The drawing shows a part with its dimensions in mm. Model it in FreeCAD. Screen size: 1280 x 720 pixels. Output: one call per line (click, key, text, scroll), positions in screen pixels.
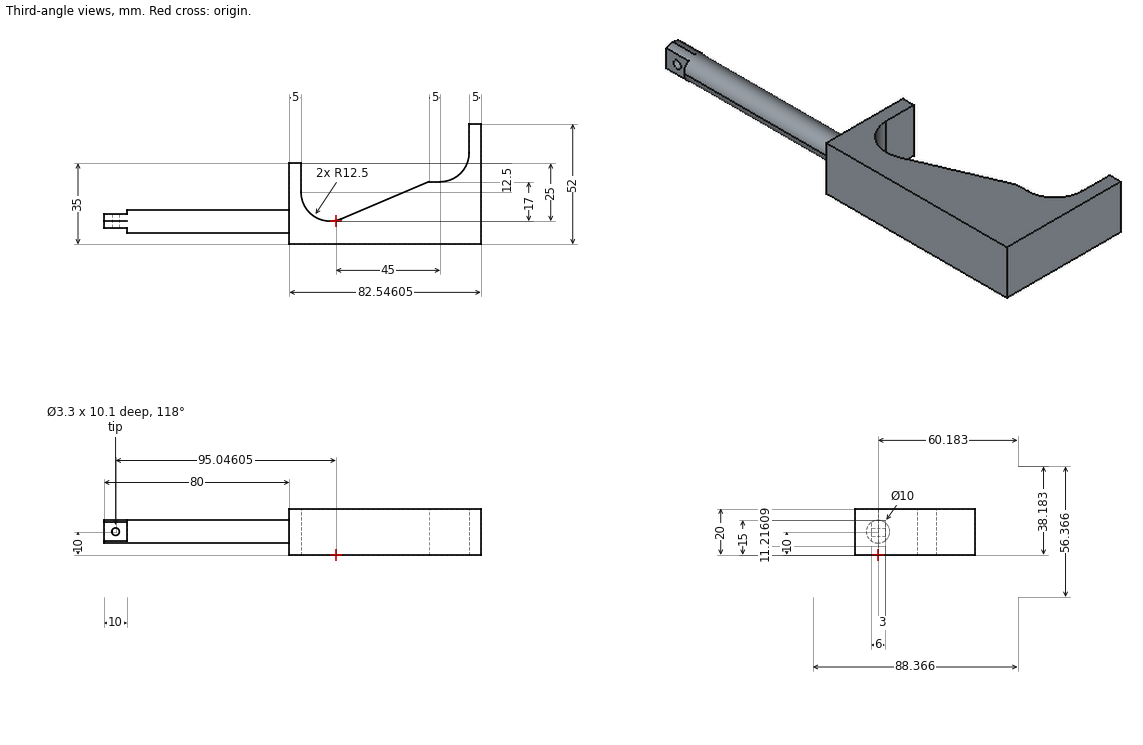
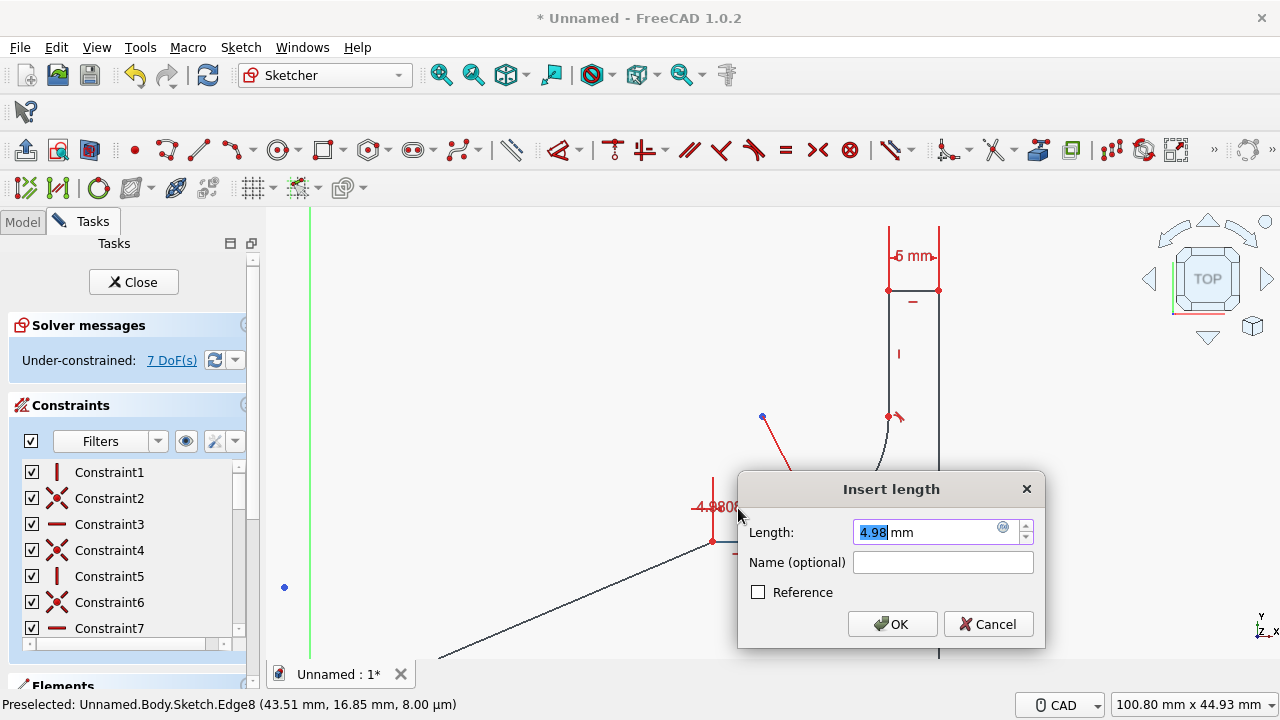
text(5)
key(Return)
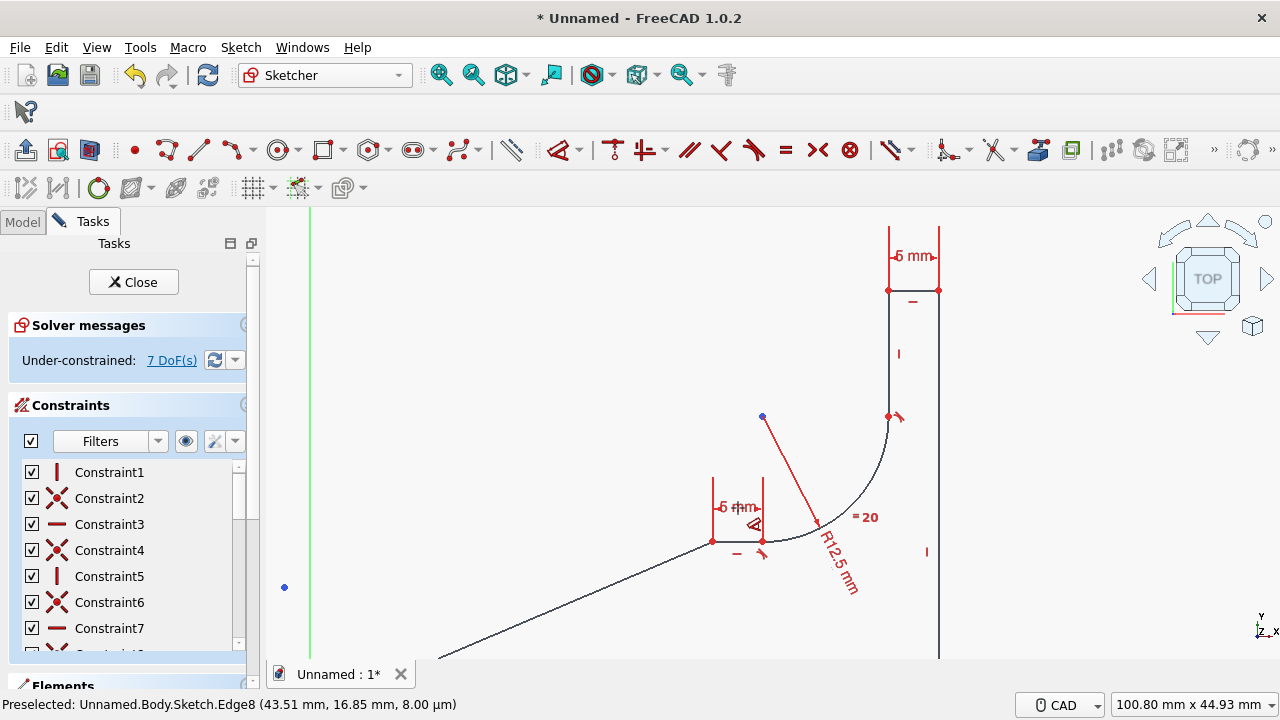
scroll(924, 290, down, 3)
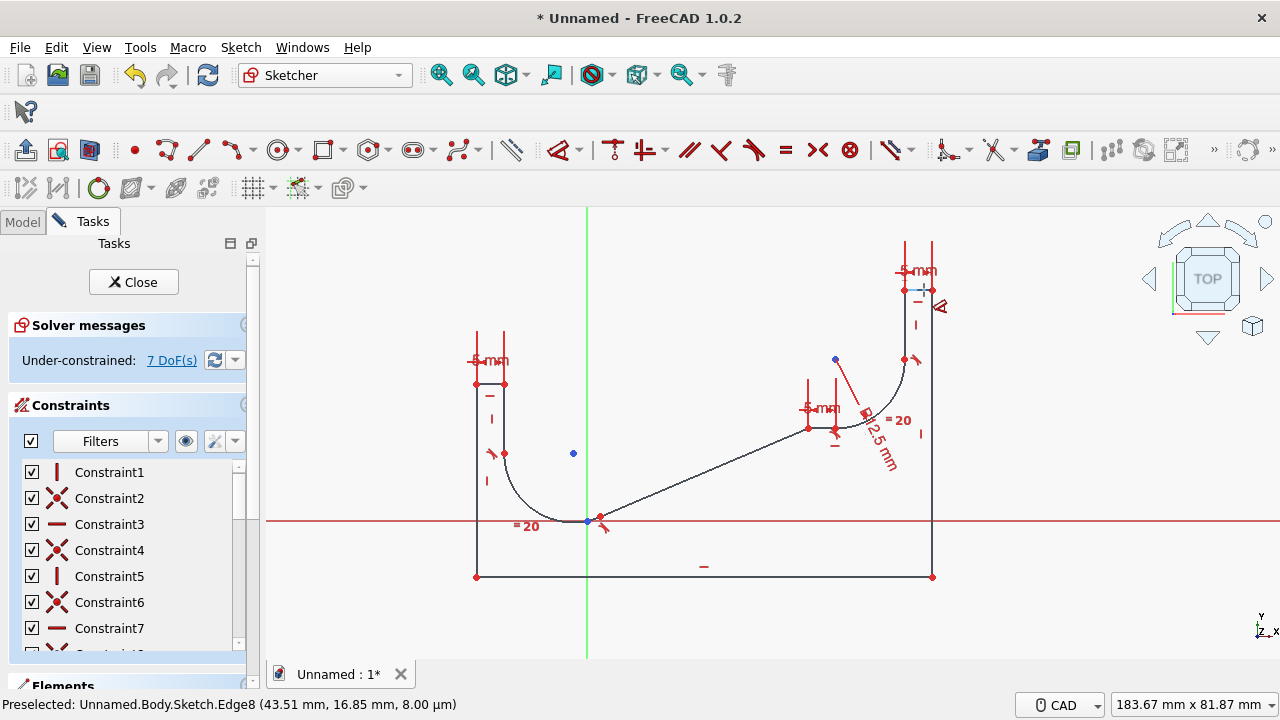
click(477, 442)
click(443, 481)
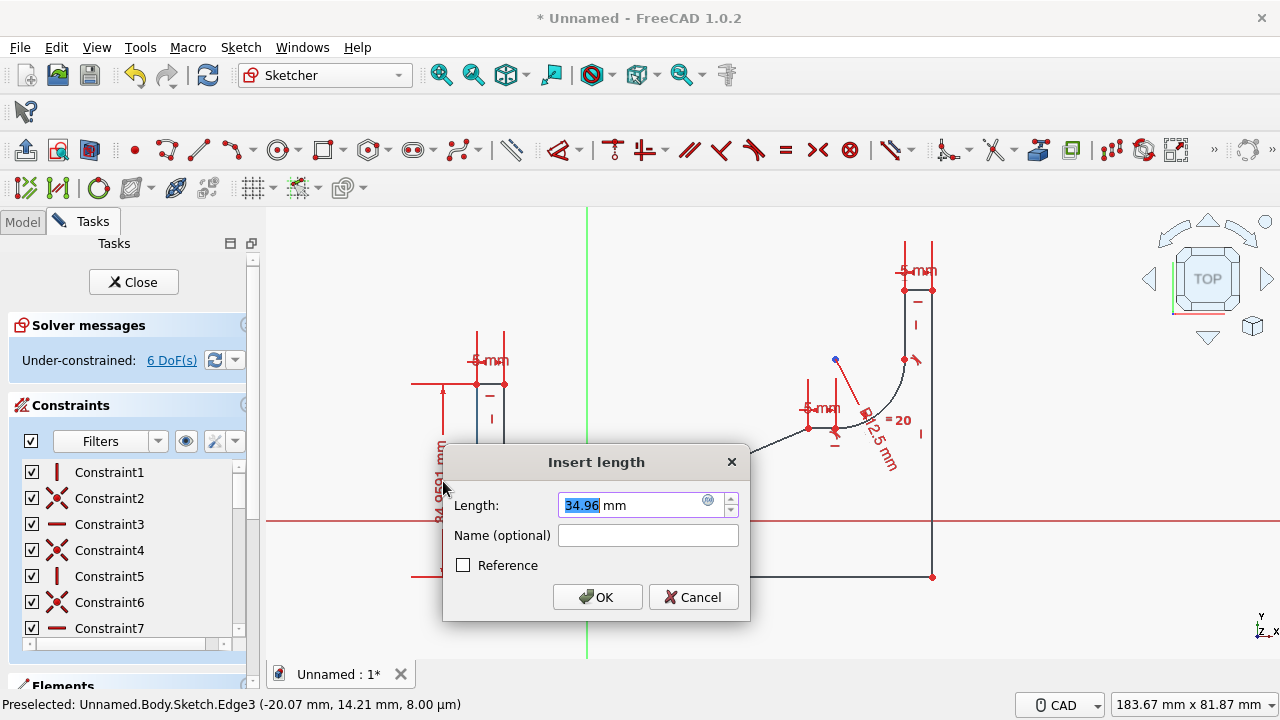
text(35)
key(Return)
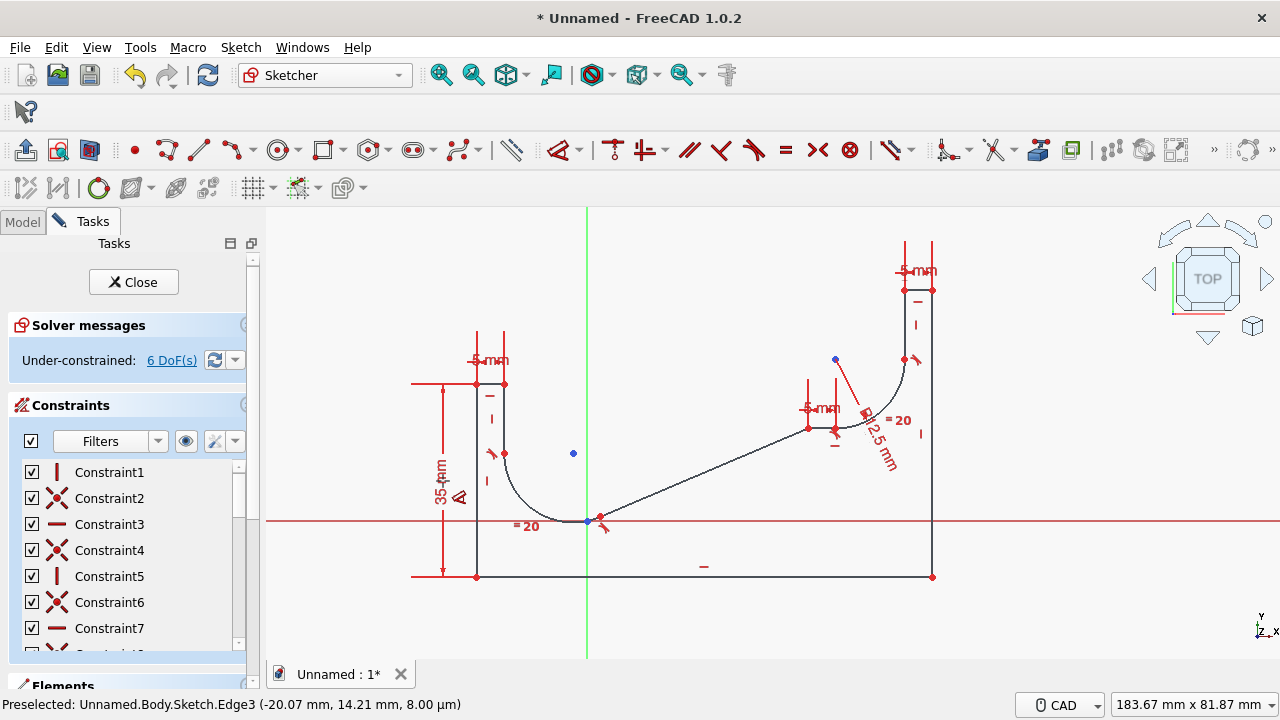
click(932, 491)
click(966, 434)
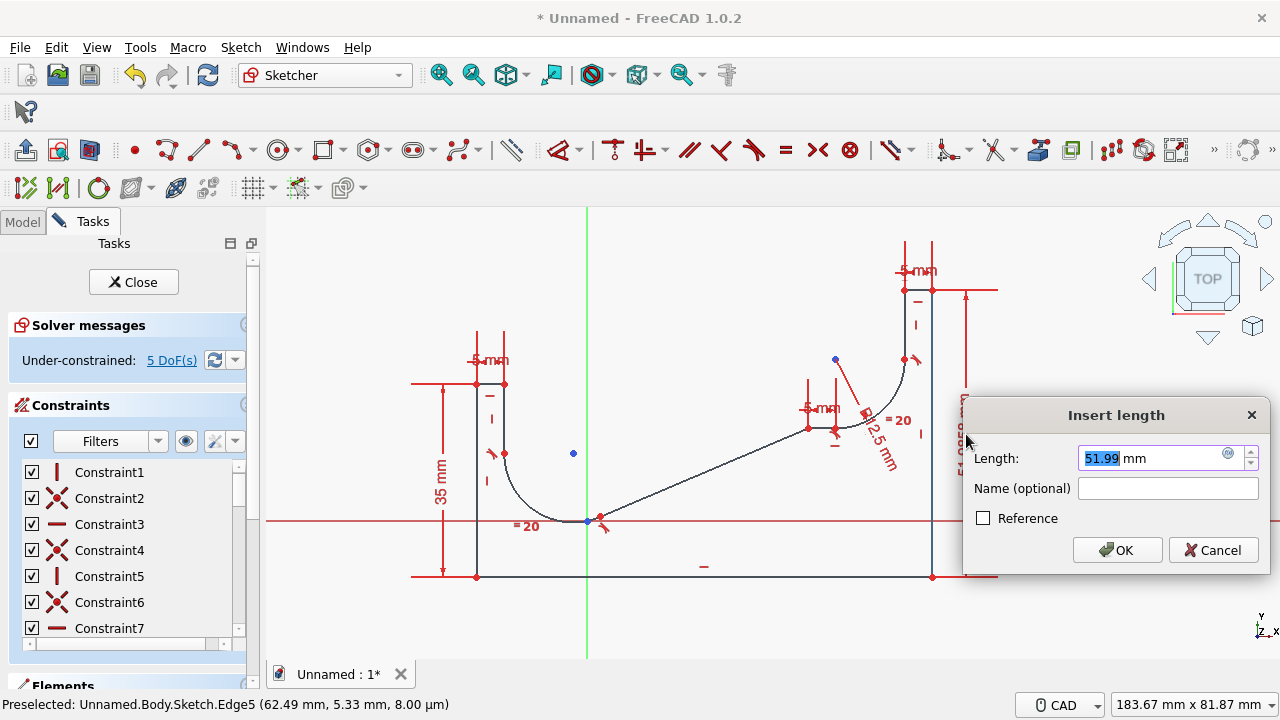
text(52)
key(Return)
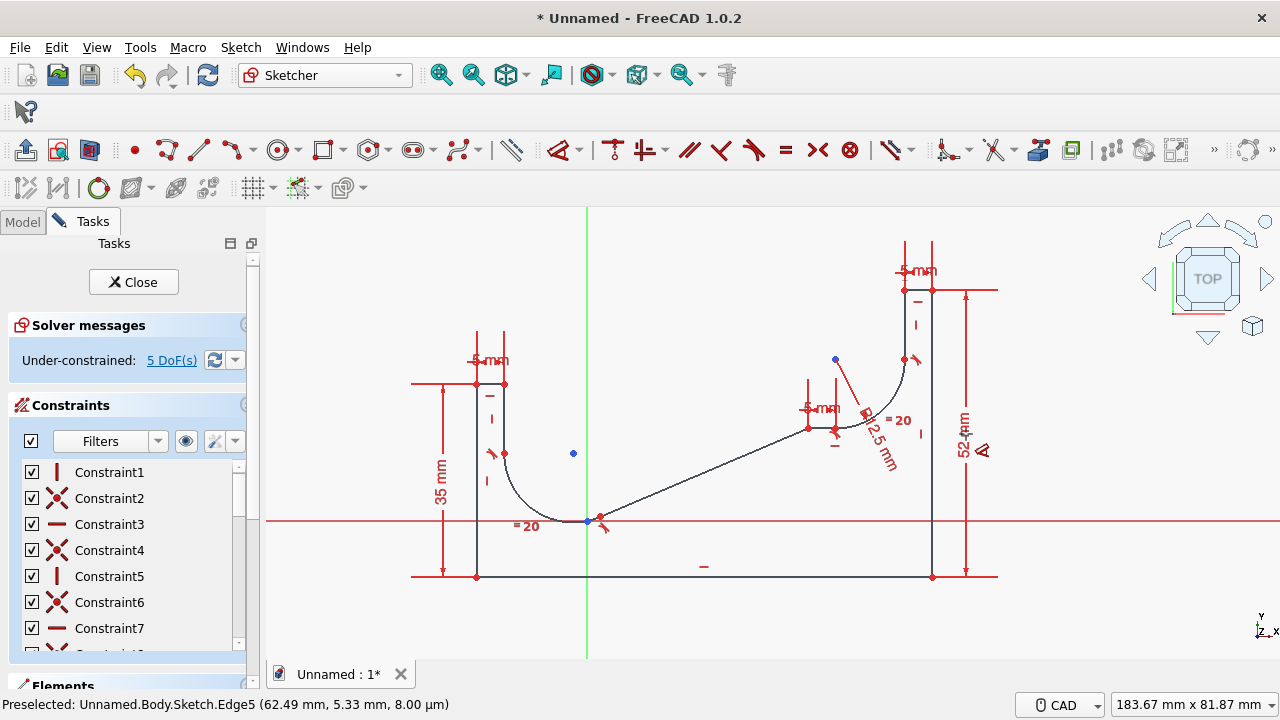
click(504, 384)
click(621, 453)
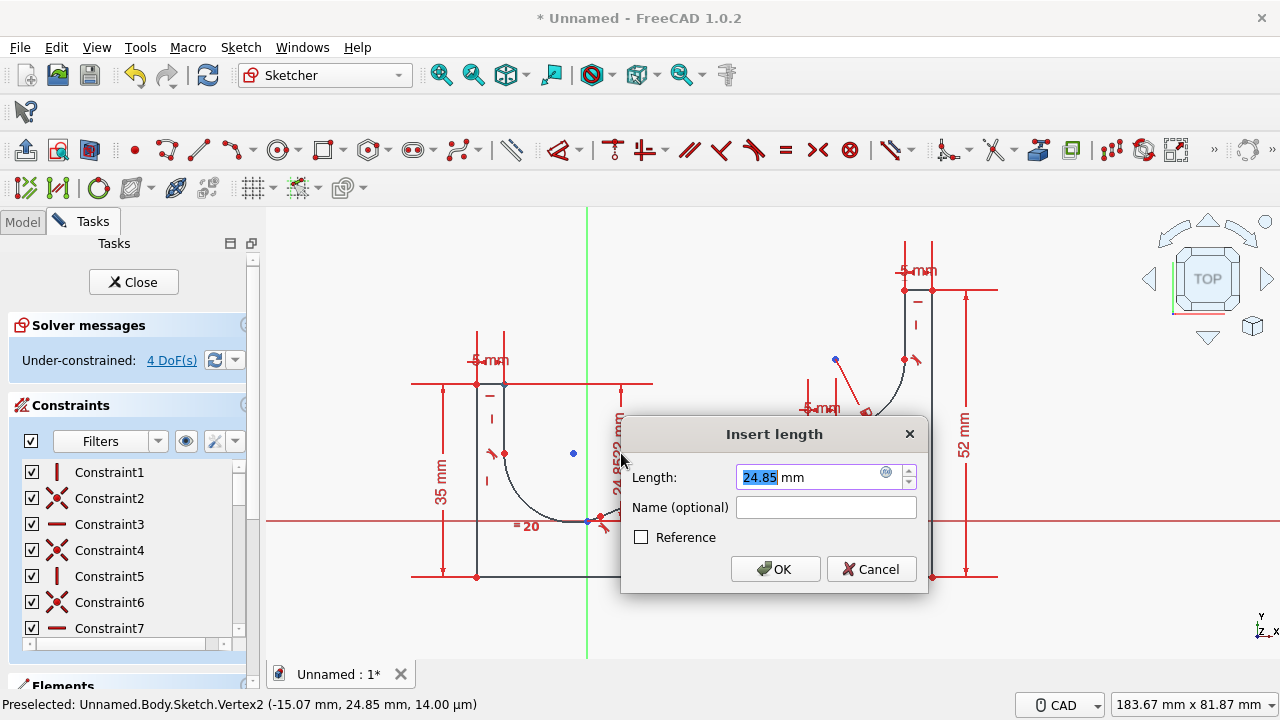
text(25)
key(Return)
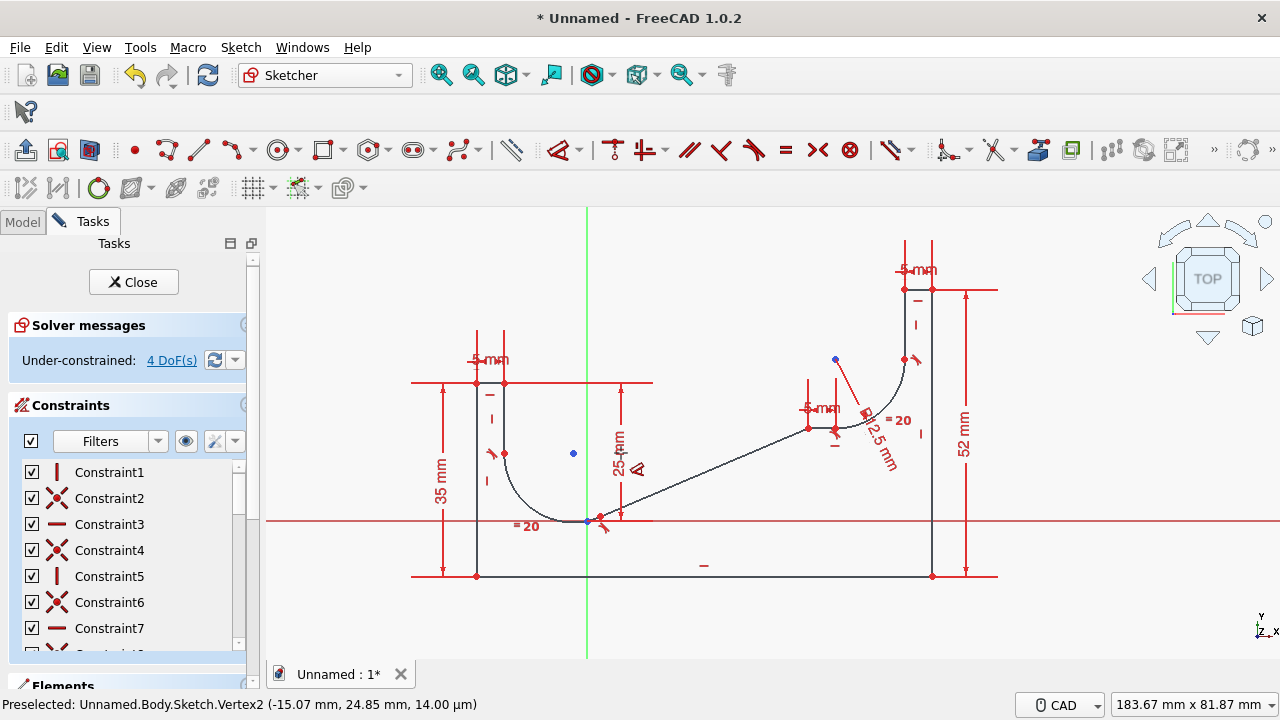
click(836, 428)
click(712, 555)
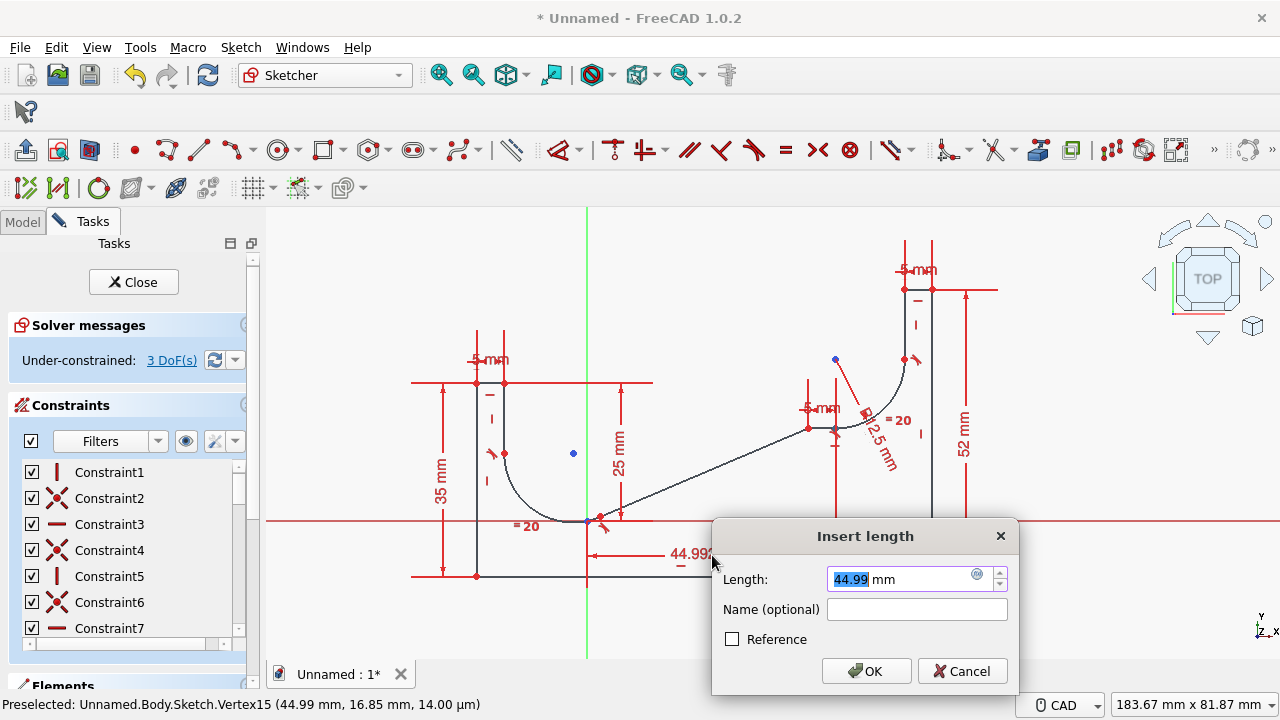
text(45)
key(Return)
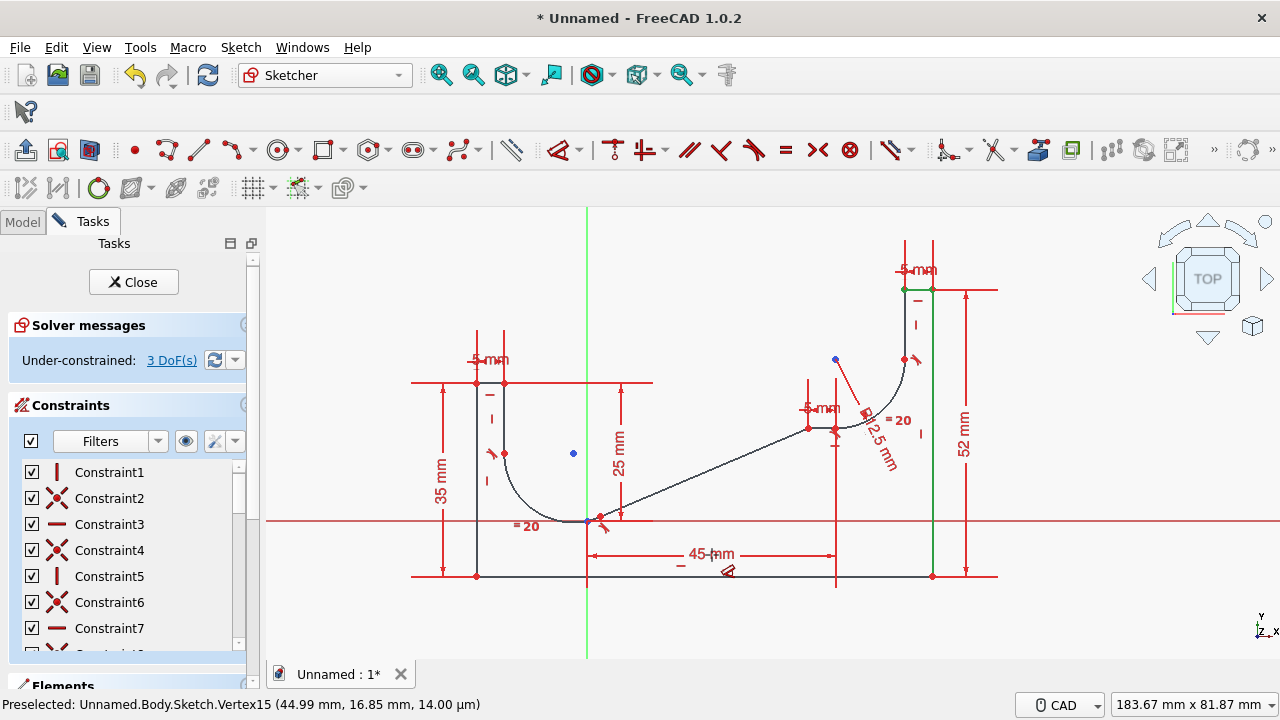
click(836, 428)
click(870, 475)